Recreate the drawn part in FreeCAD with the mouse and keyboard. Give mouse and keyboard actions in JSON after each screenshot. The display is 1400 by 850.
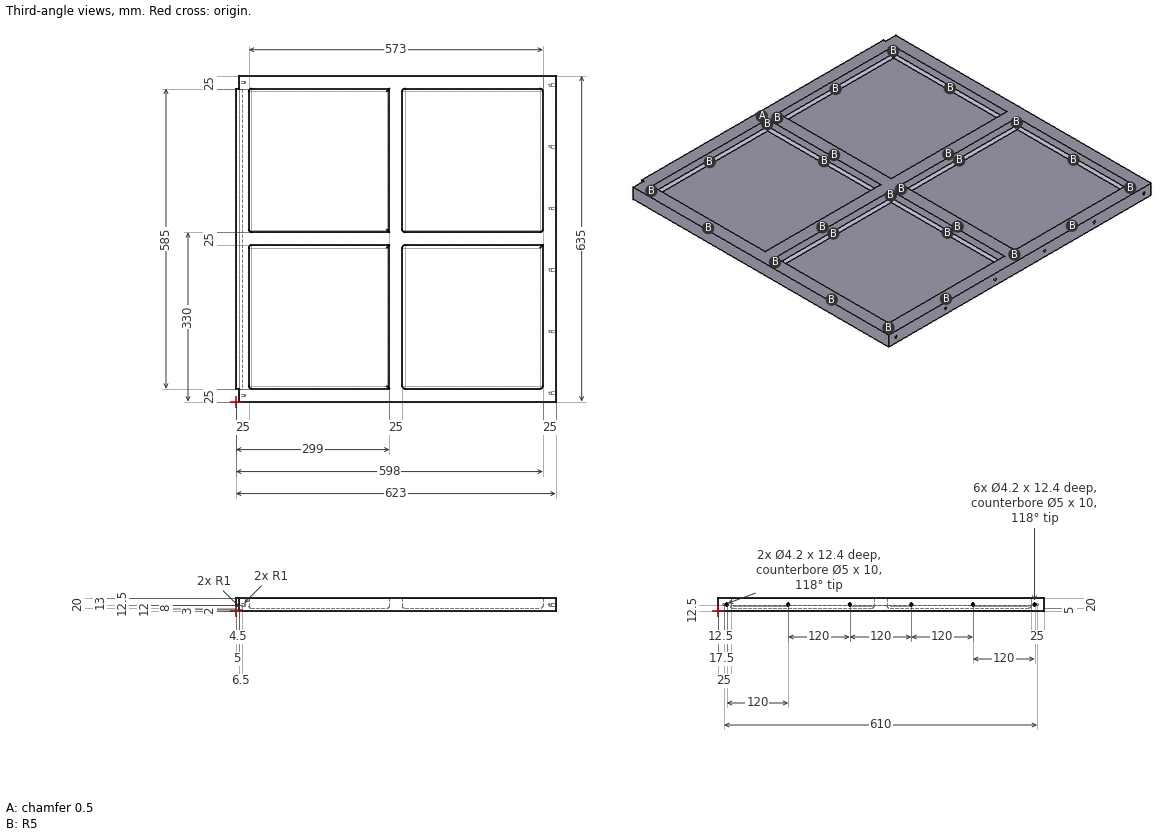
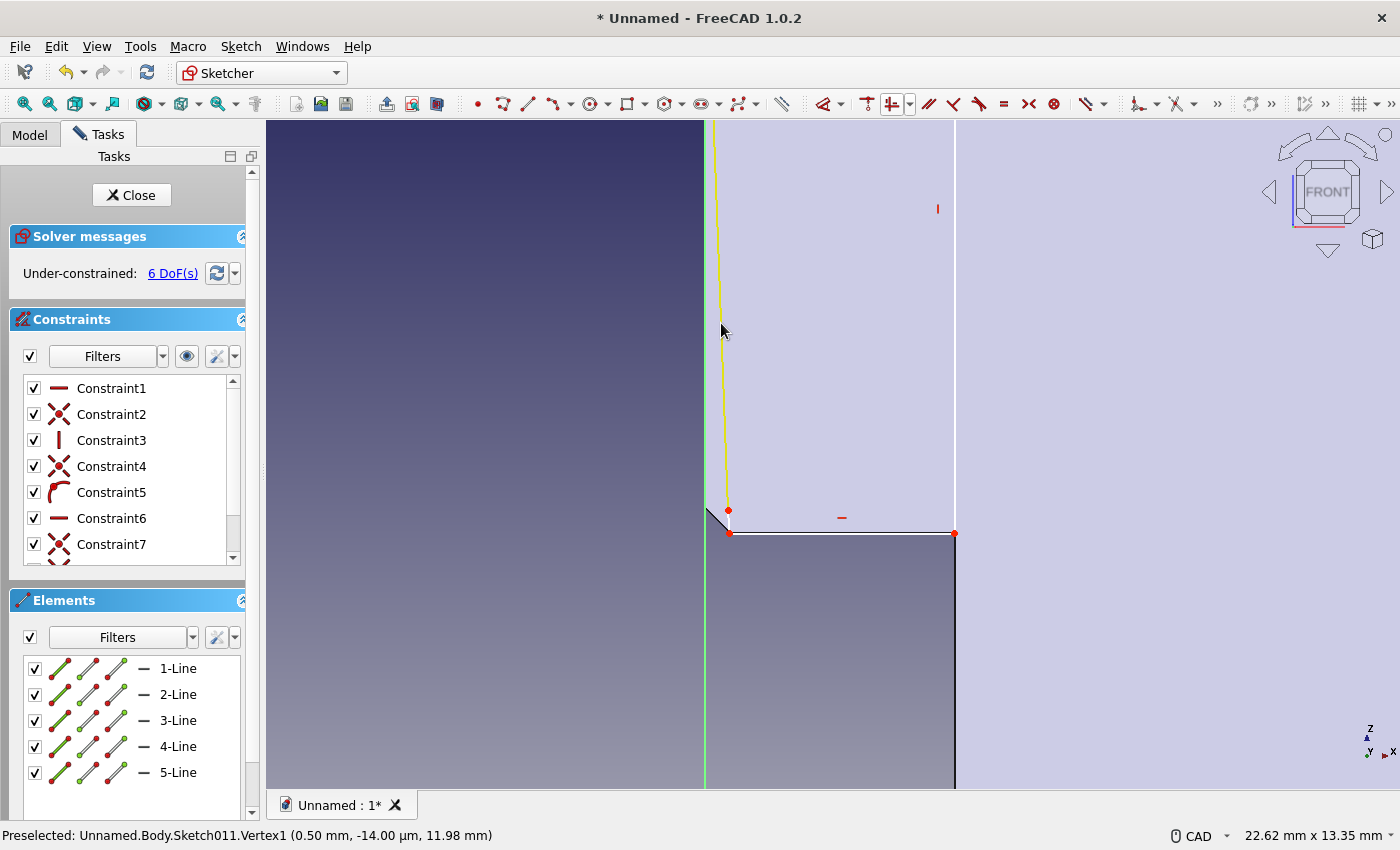
{"action": "left_click", "coordinate": [721, 322]}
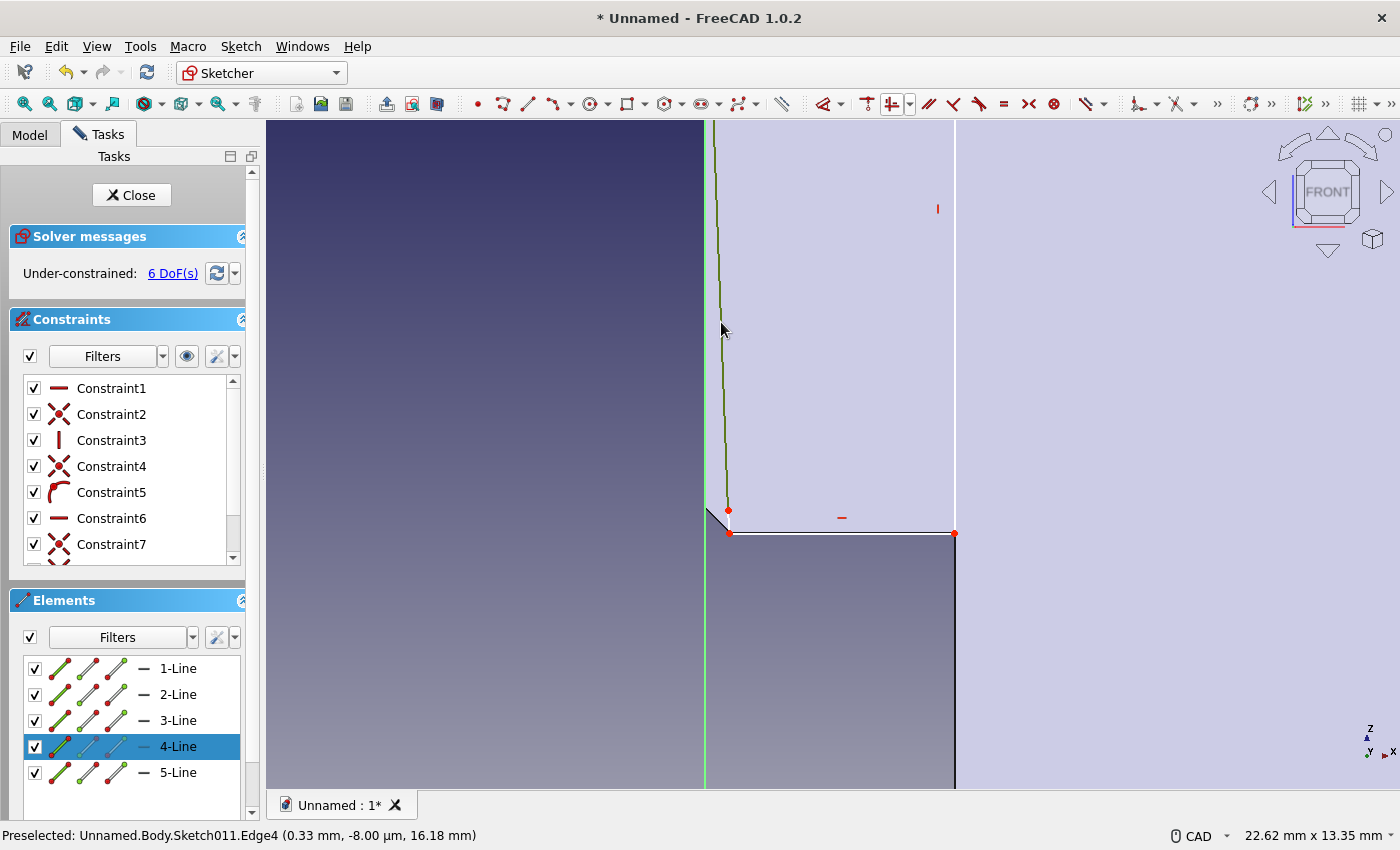
{"action": "key", "text": "v"}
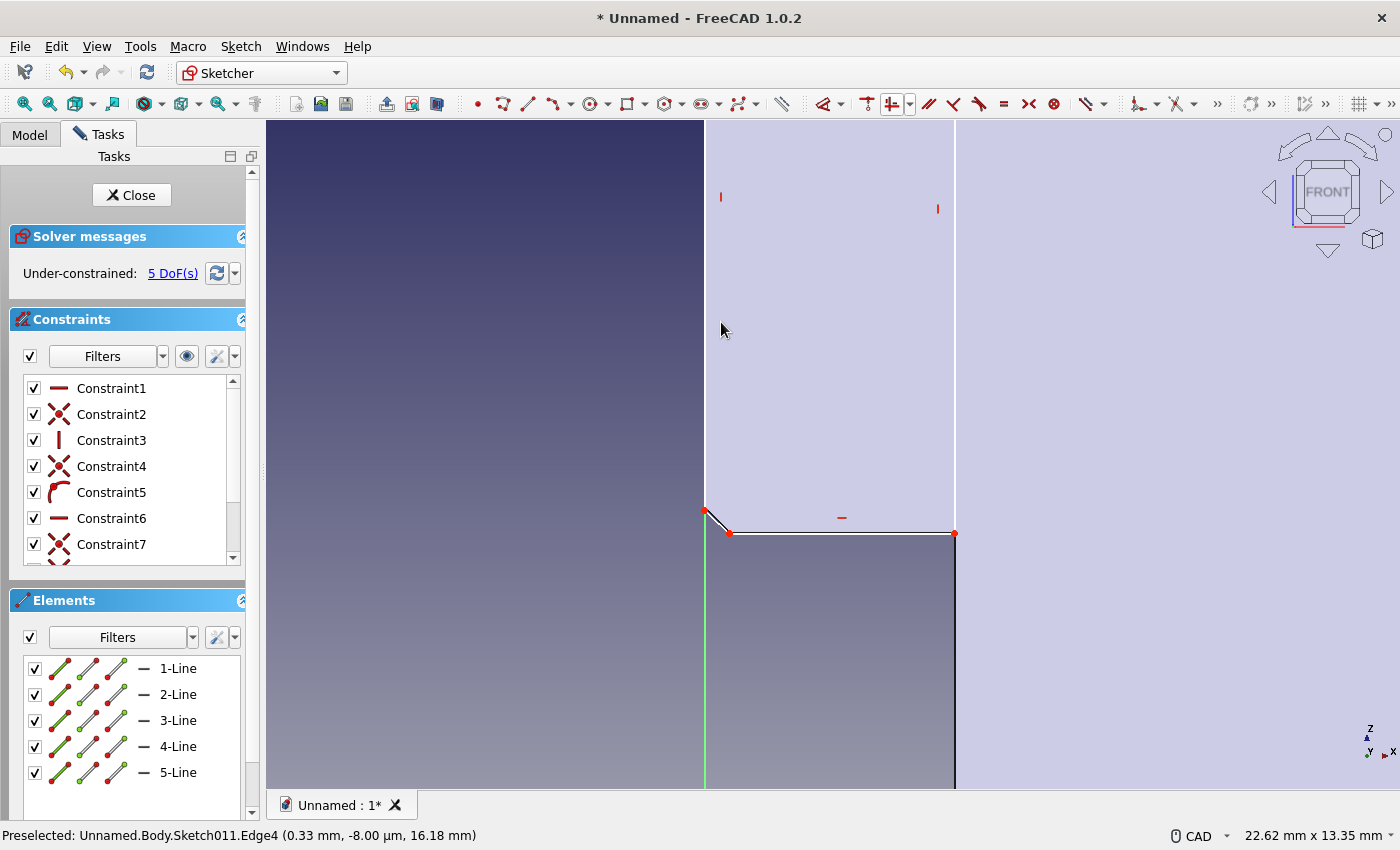
{"action": "left_click", "coordinate": [822, 104]}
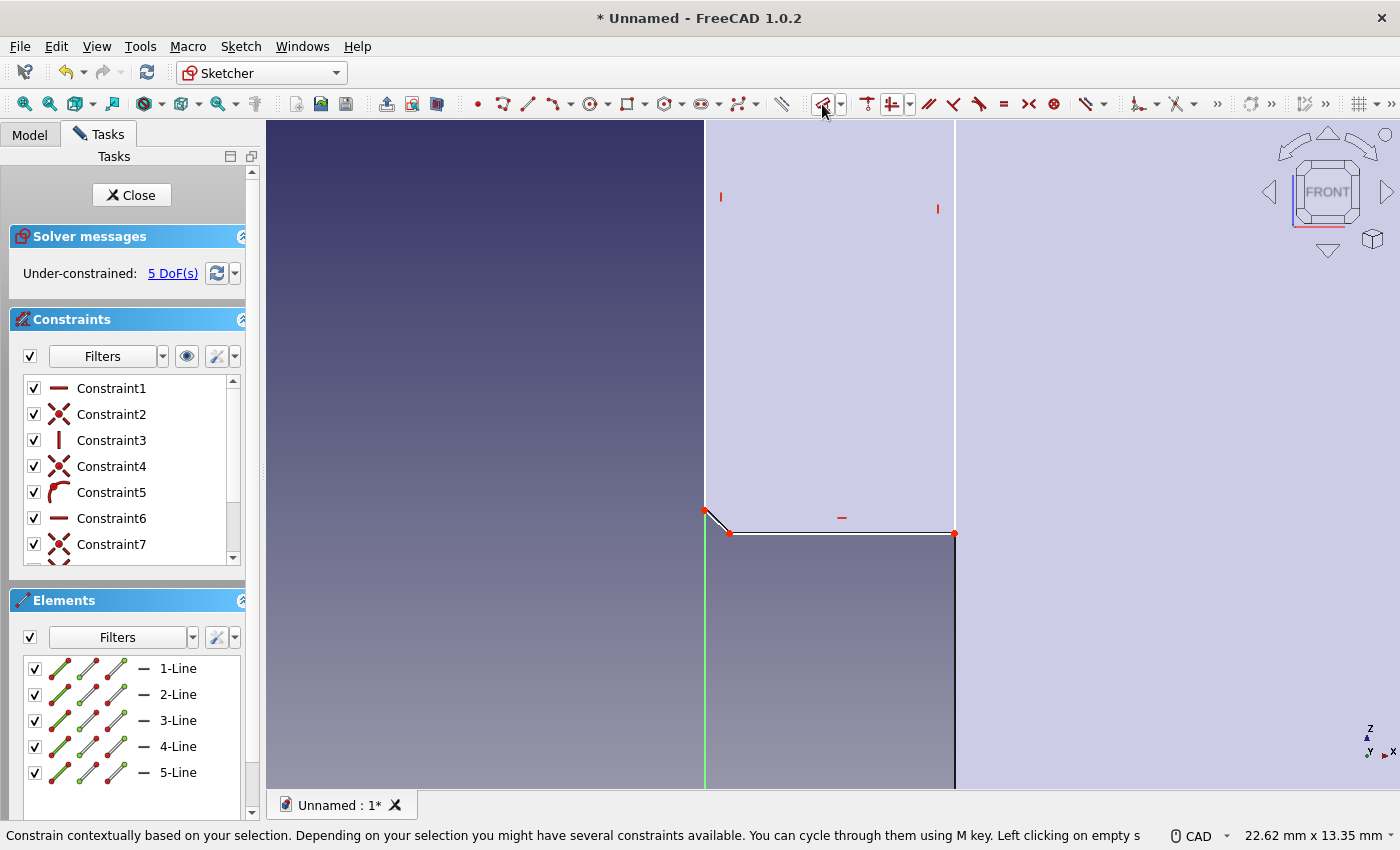
{"action": "scroll", "coordinate": [726, 424], "scroll_direction": "down", "scroll_amount": 5}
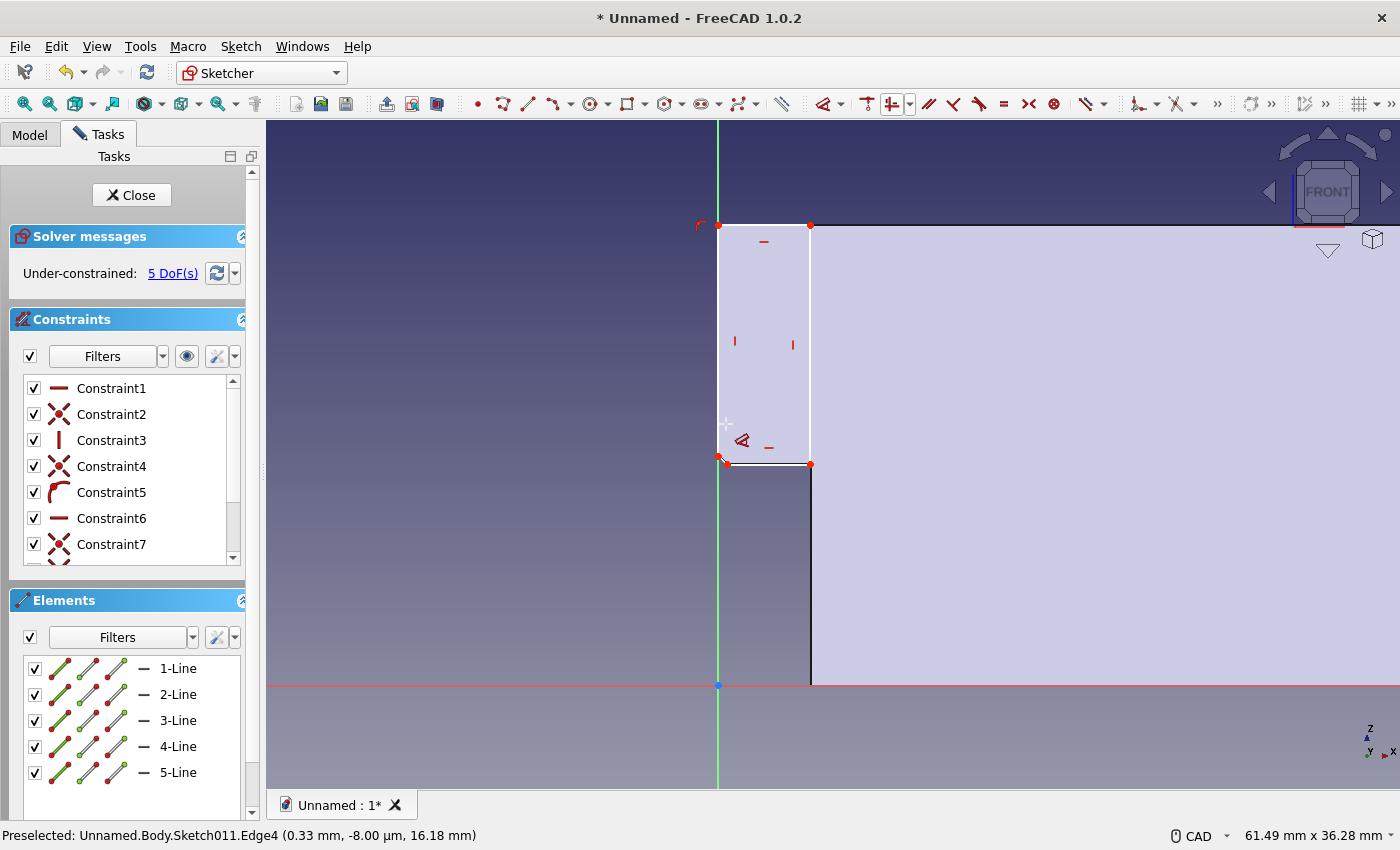
{"action": "left_click", "coordinate": [783, 225]}
{"action": "left_click", "coordinate": [764, 191]}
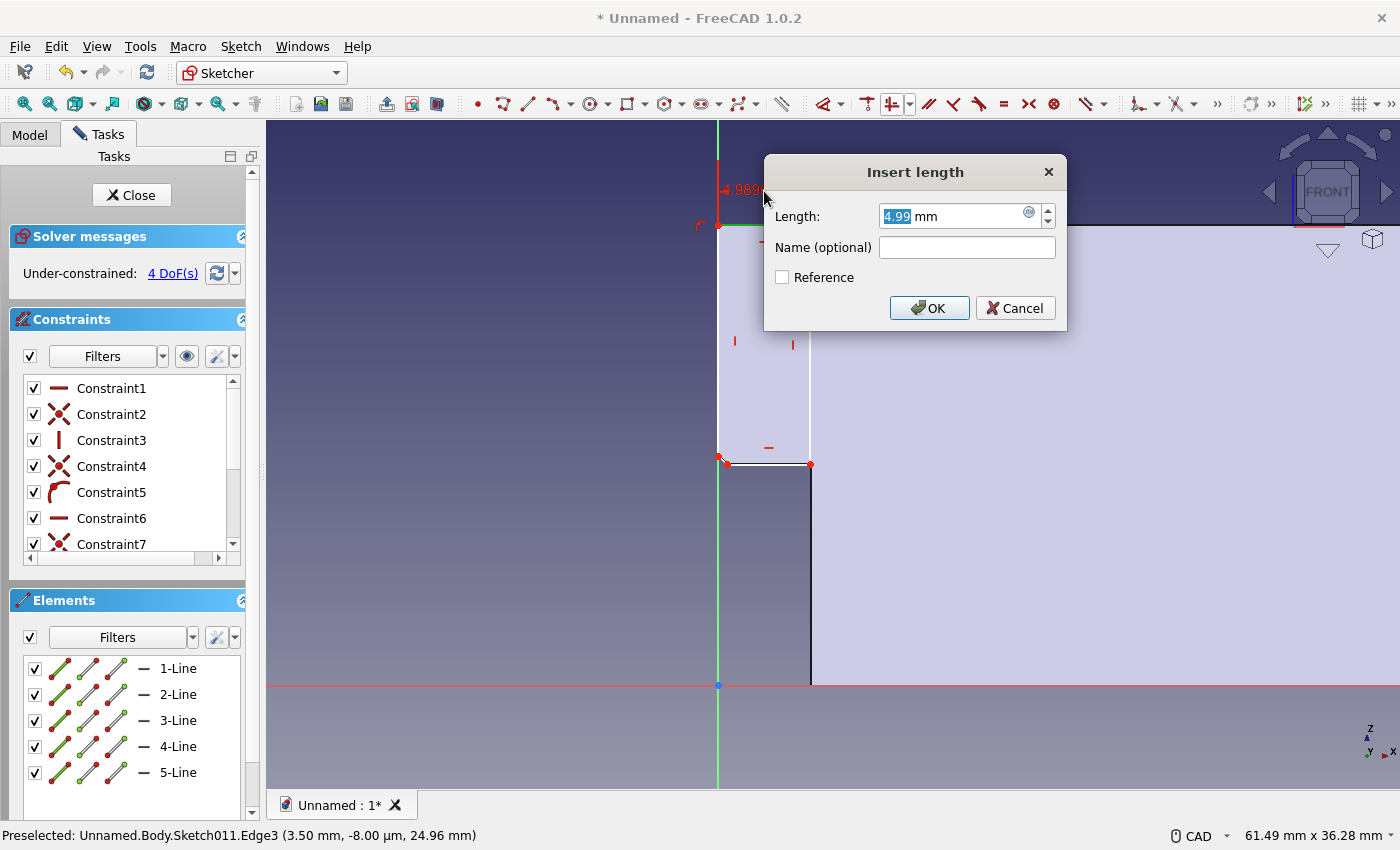
{"action": "type", "text": "5"}
{"action": "key", "text": "Return"}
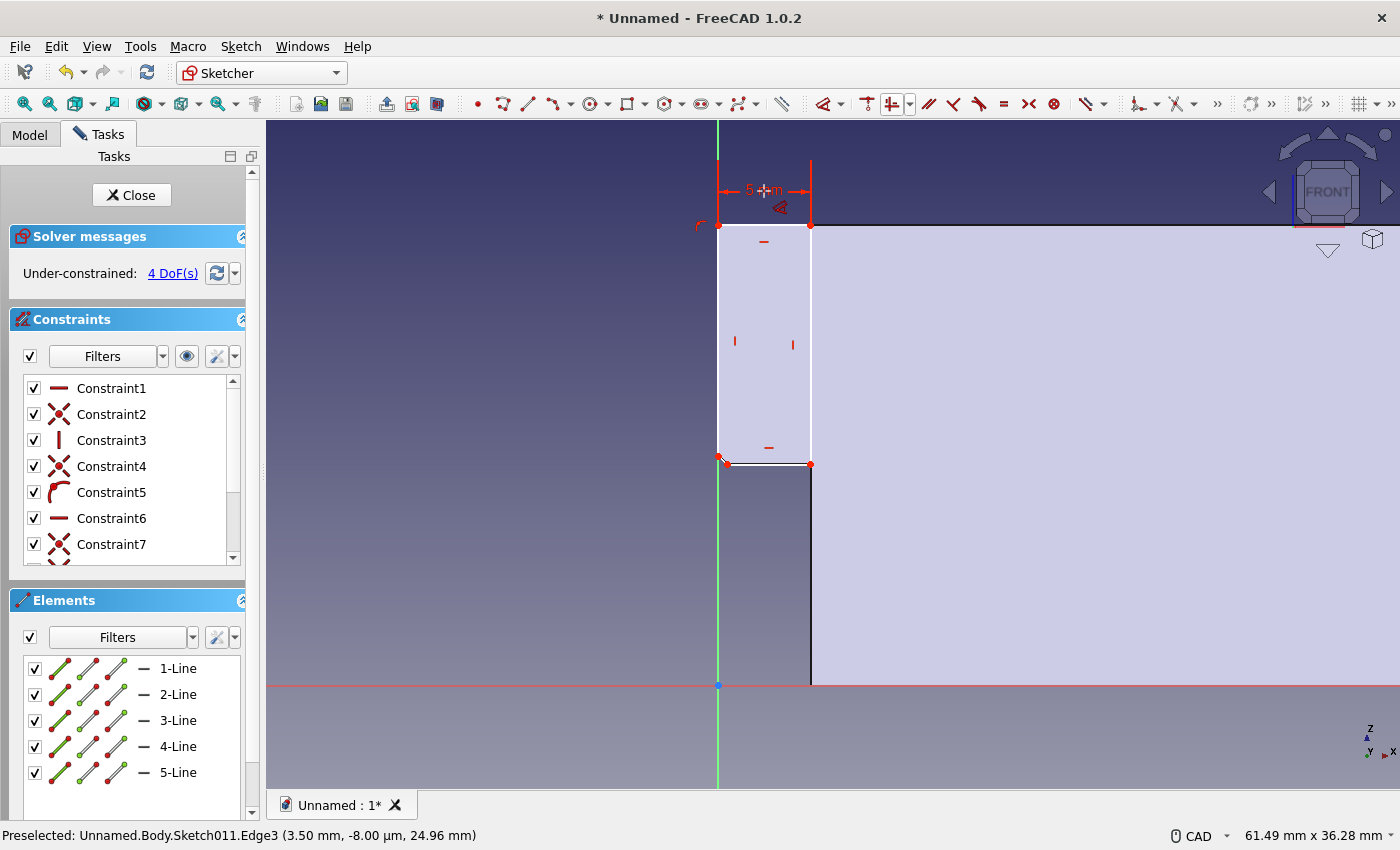
{"action": "left_click", "coordinate": [811, 393]}
{"action": "left_click", "coordinate": [845, 345]}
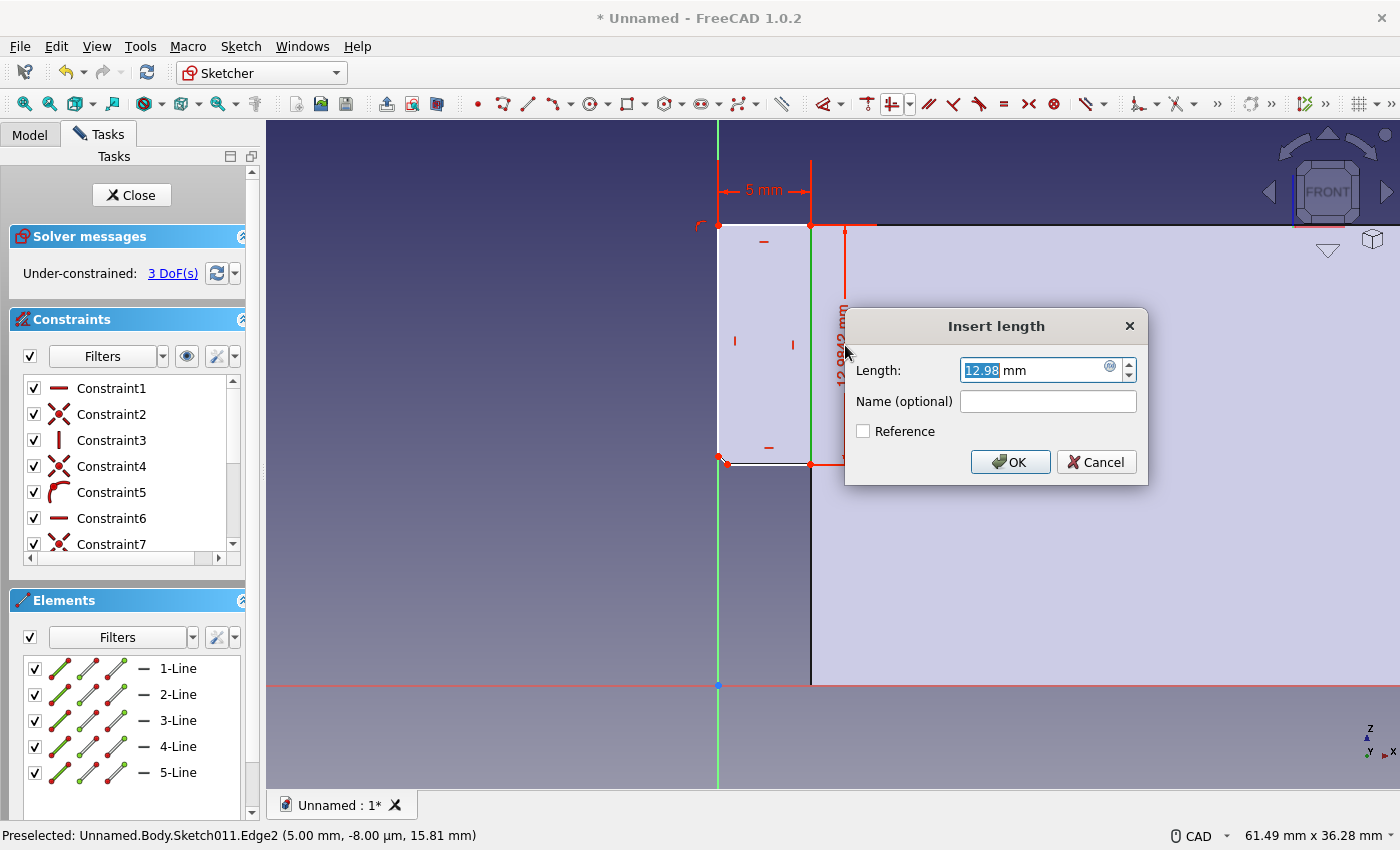
{"action": "type", "text": "13"}
{"action": "key", "text": "Return"}